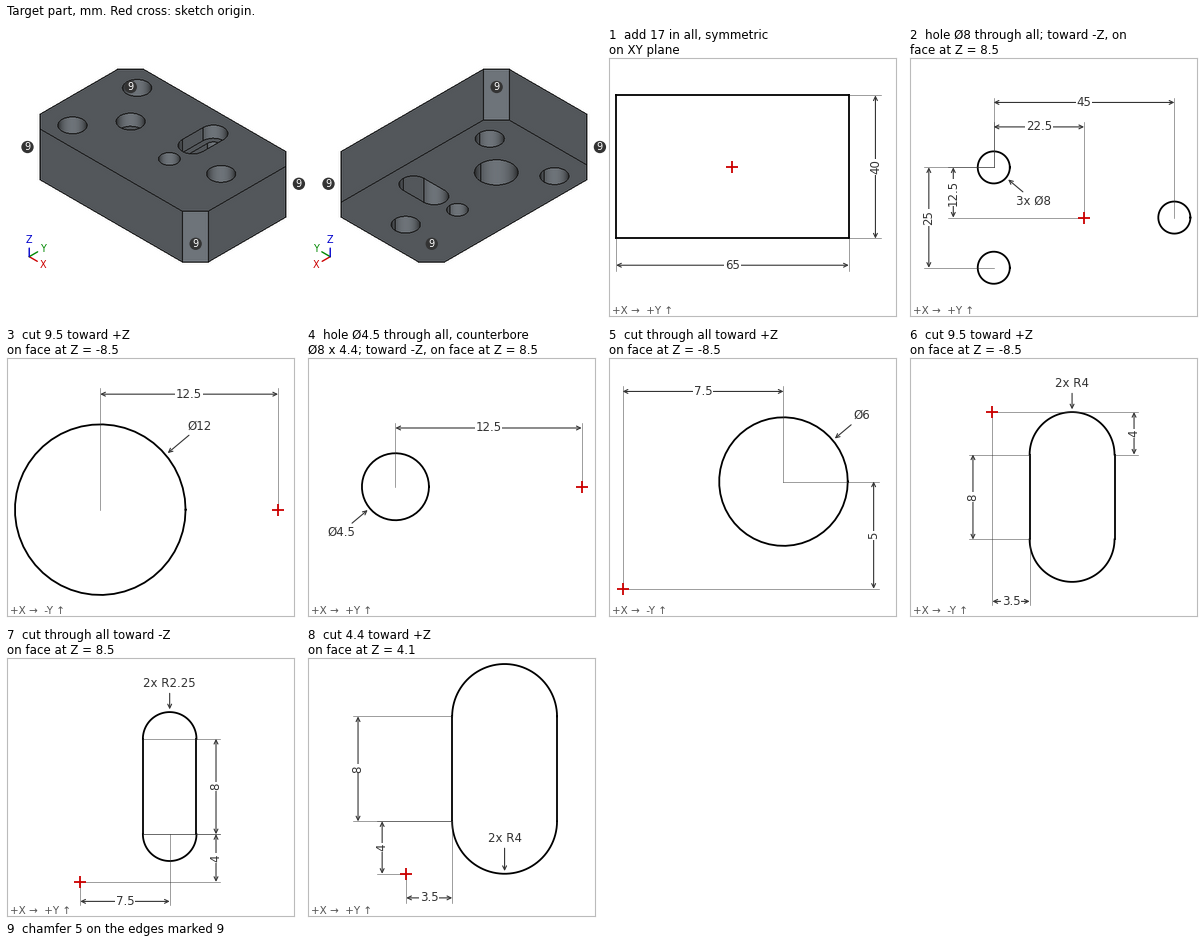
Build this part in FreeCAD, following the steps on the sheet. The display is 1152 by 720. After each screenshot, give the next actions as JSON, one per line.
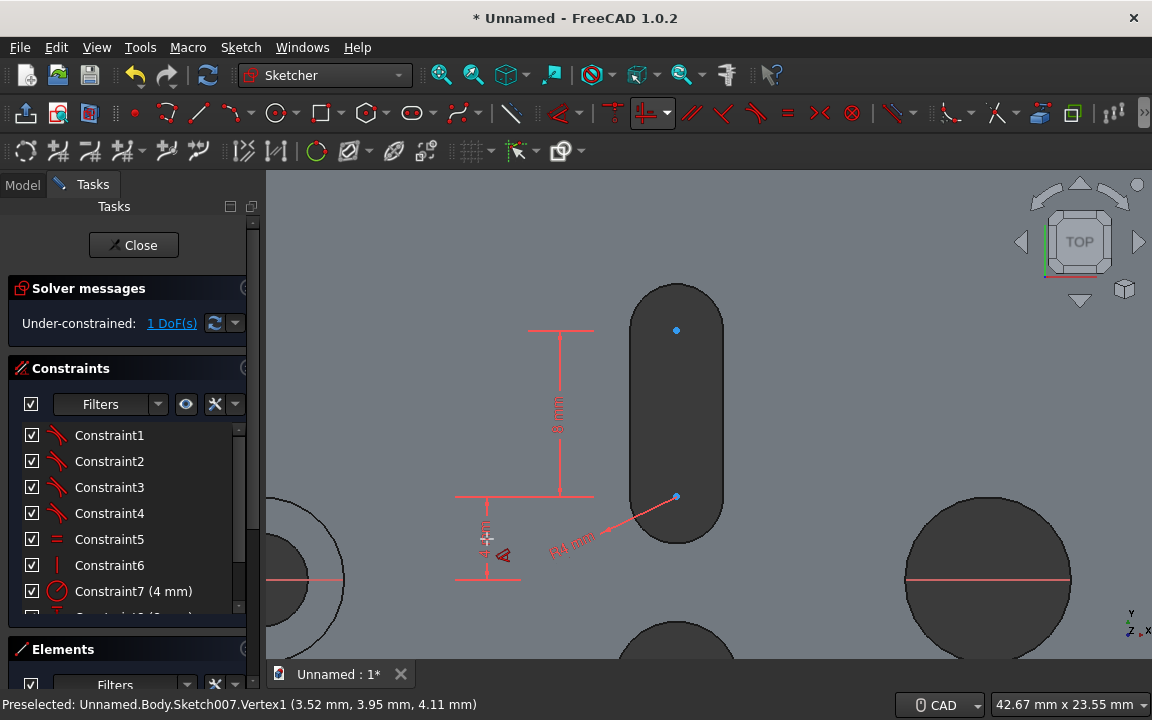
{"action": "left_click", "coordinate": [594, 497]}
{"action": "left_click", "coordinate": [557, 614]}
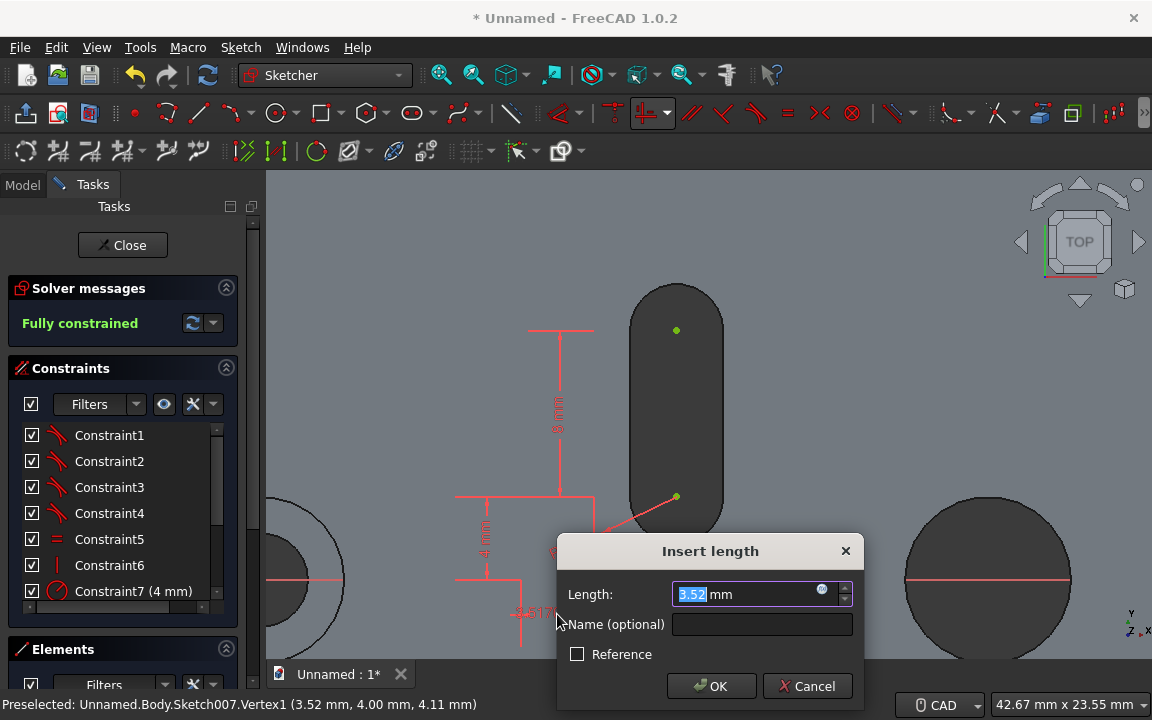
{"action": "type", "text": "3.5"}
{"action": "key", "text": "Return"}
{"action": "key", "text": "Escape"}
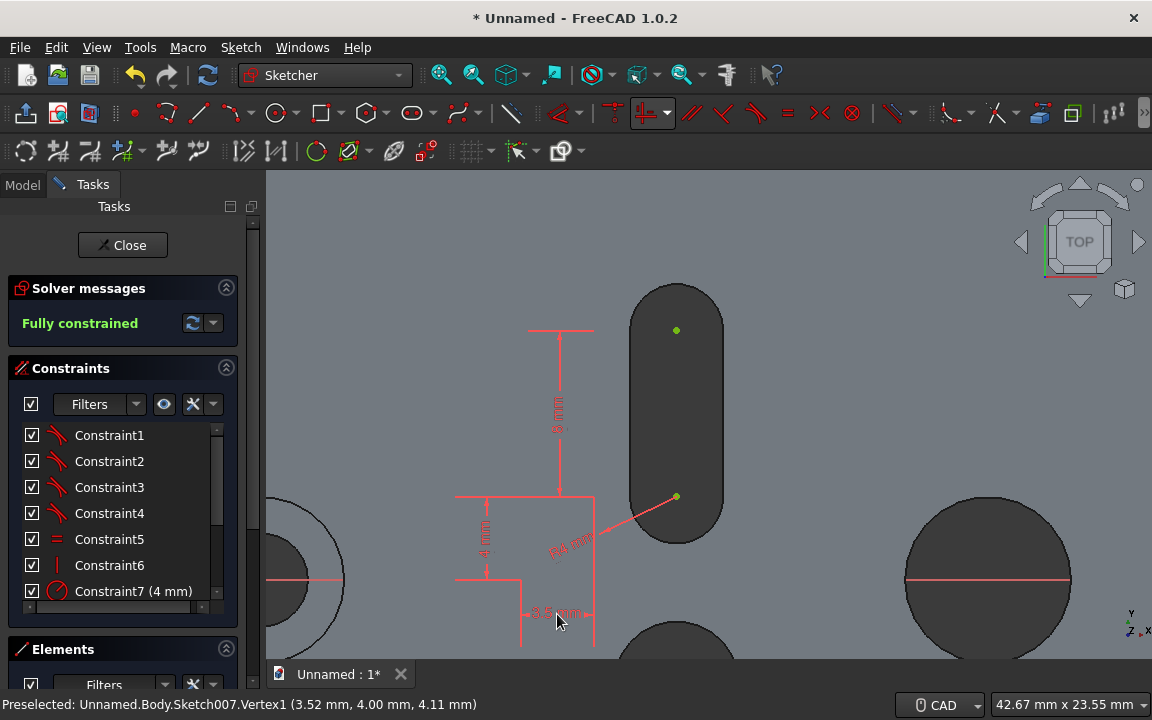
{"action": "left_click", "coordinate": [123, 245]}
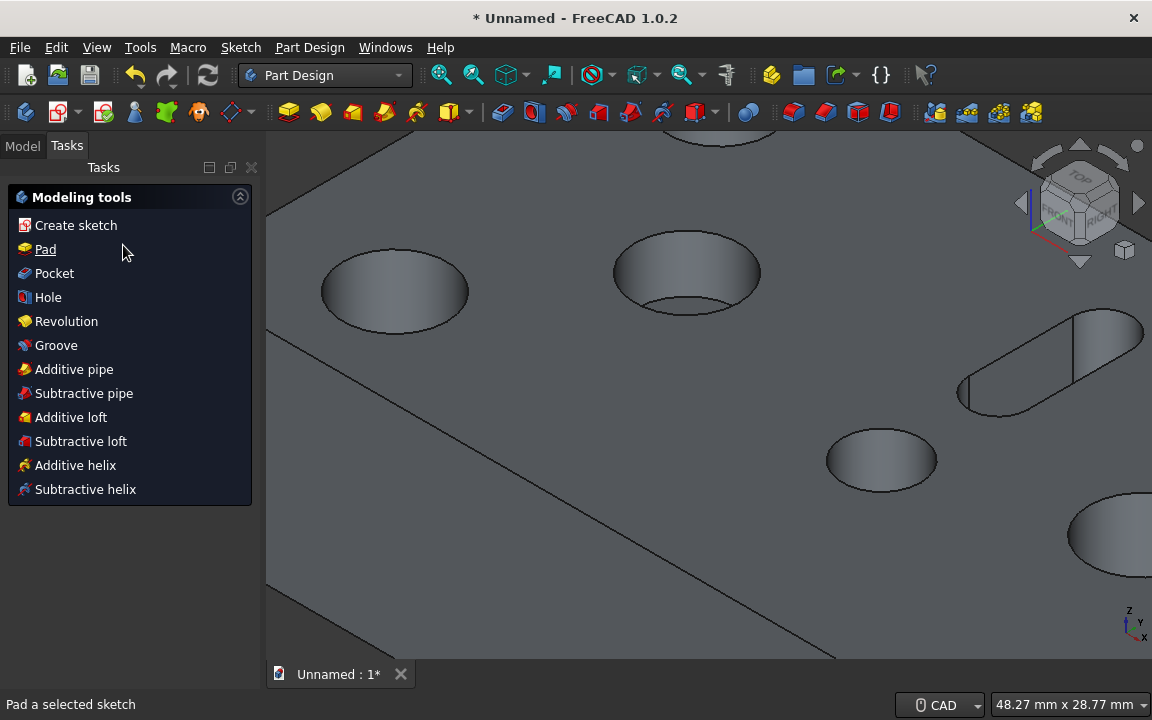
{"action": "left_click", "coordinate": [504, 112]}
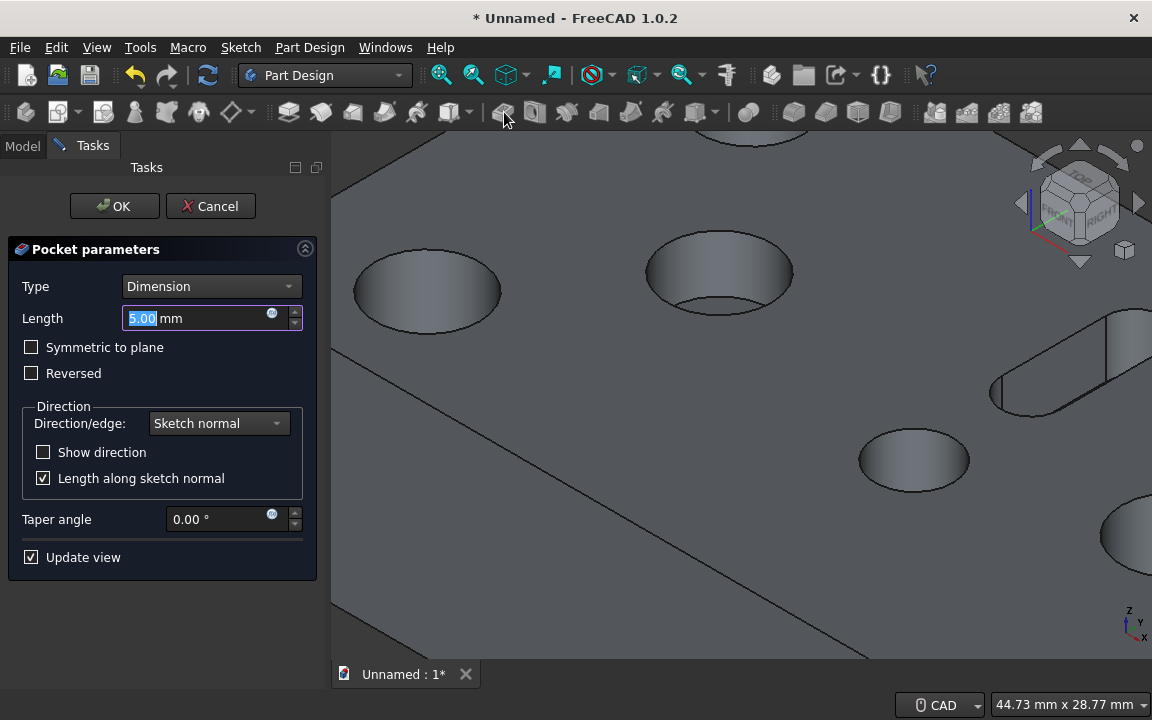
{"action": "type", "text": "4.4"}
{"action": "key", "text": "Tab"}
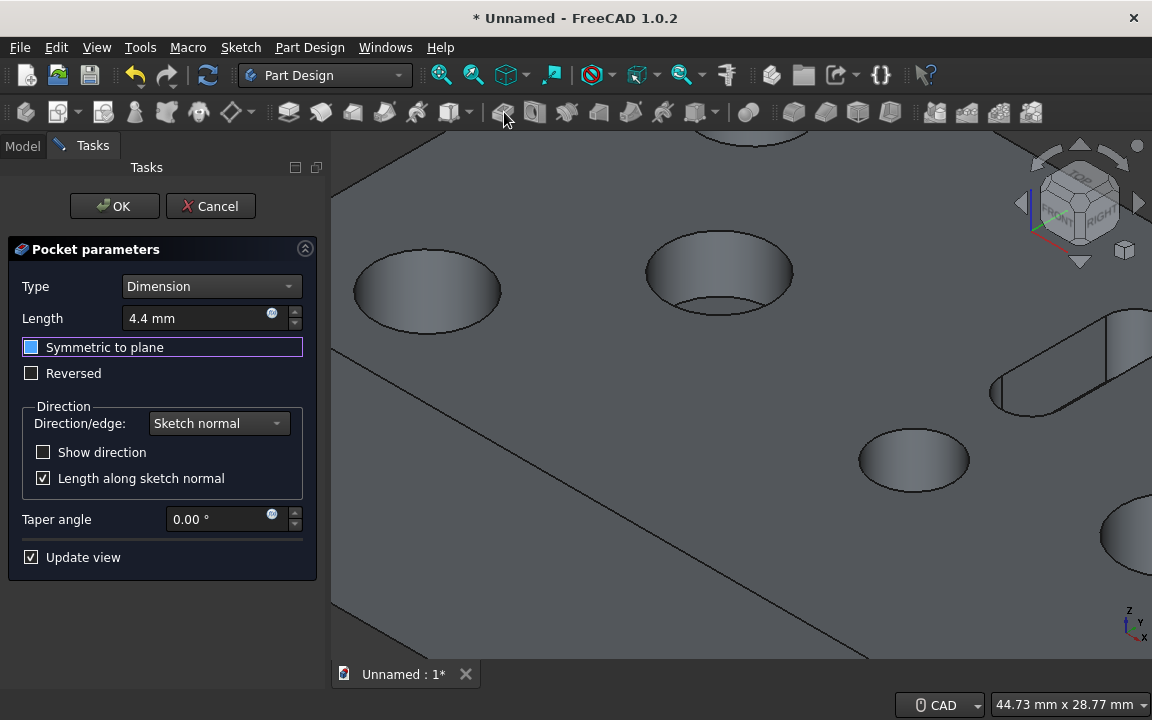
{"action": "left_click", "coordinate": [30, 373]}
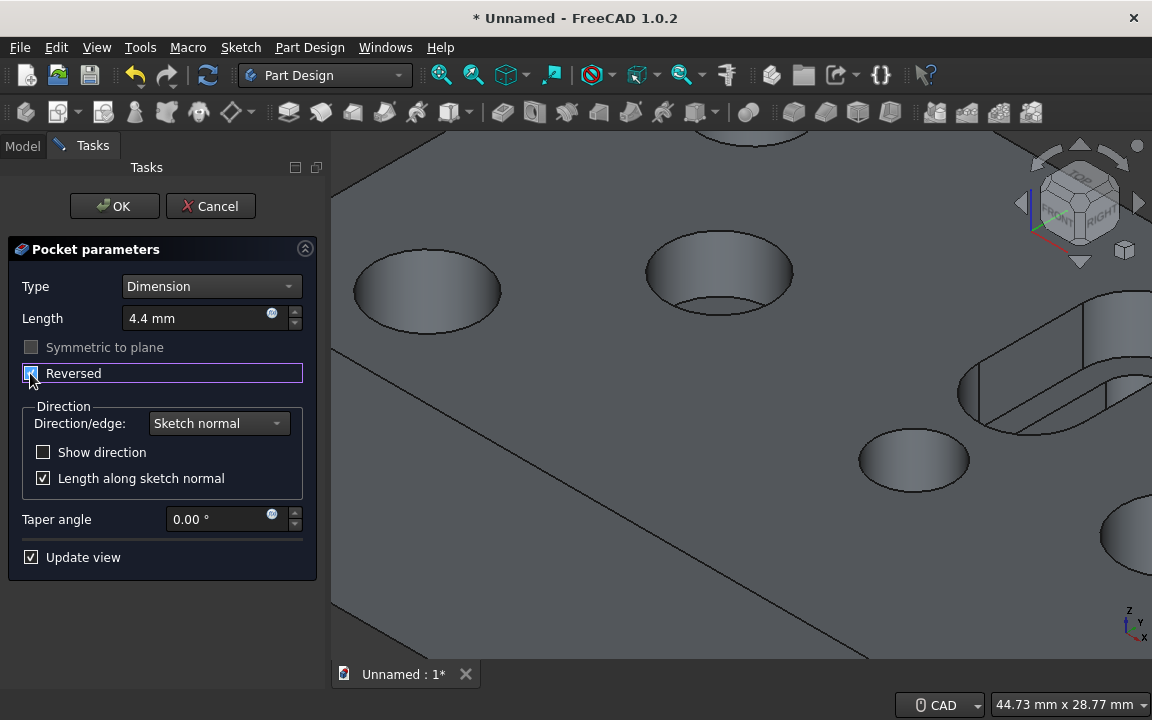
{"action": "left_click", "coordinate": [115, 206]}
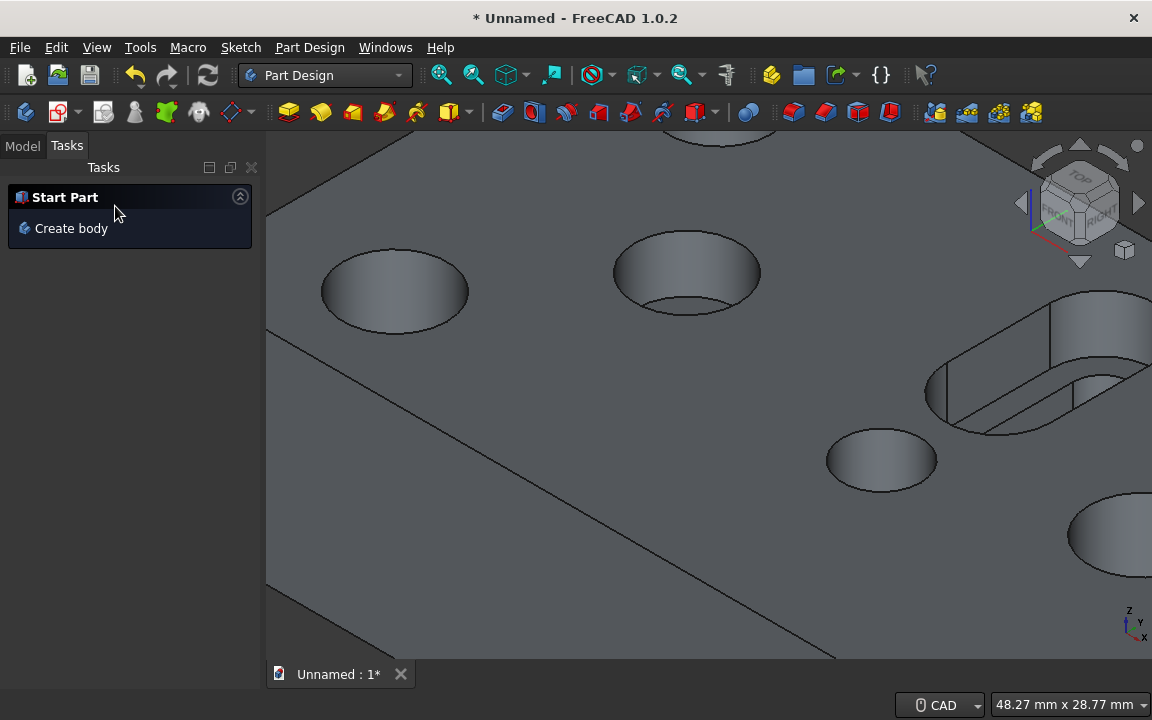
{"action": "left_click", "coordinate": [442, 76]}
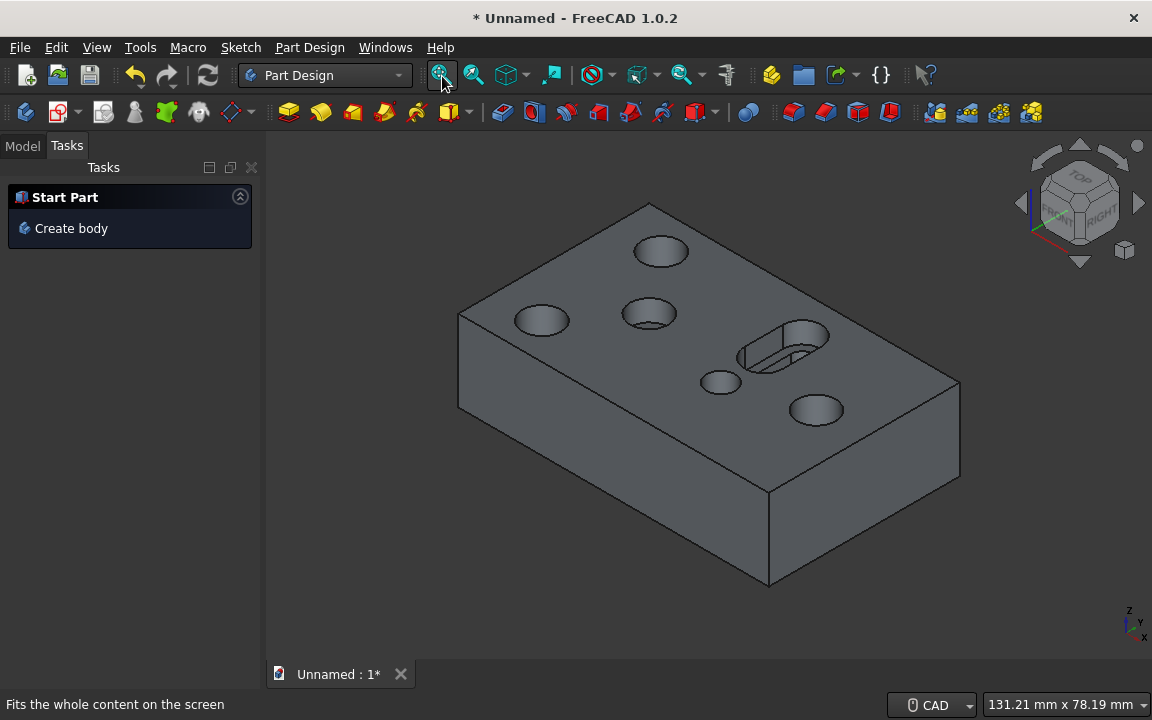
{"action": "left_click", "coordinate": [769, 539]}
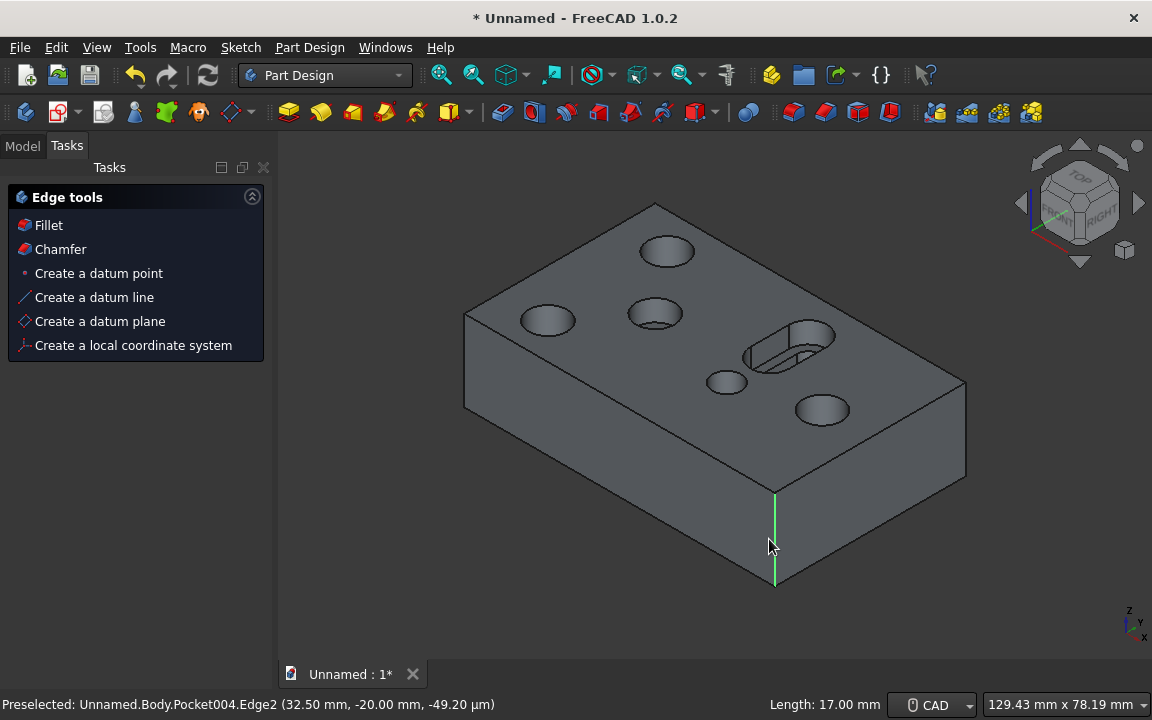
{"action": "key", "text": "2"}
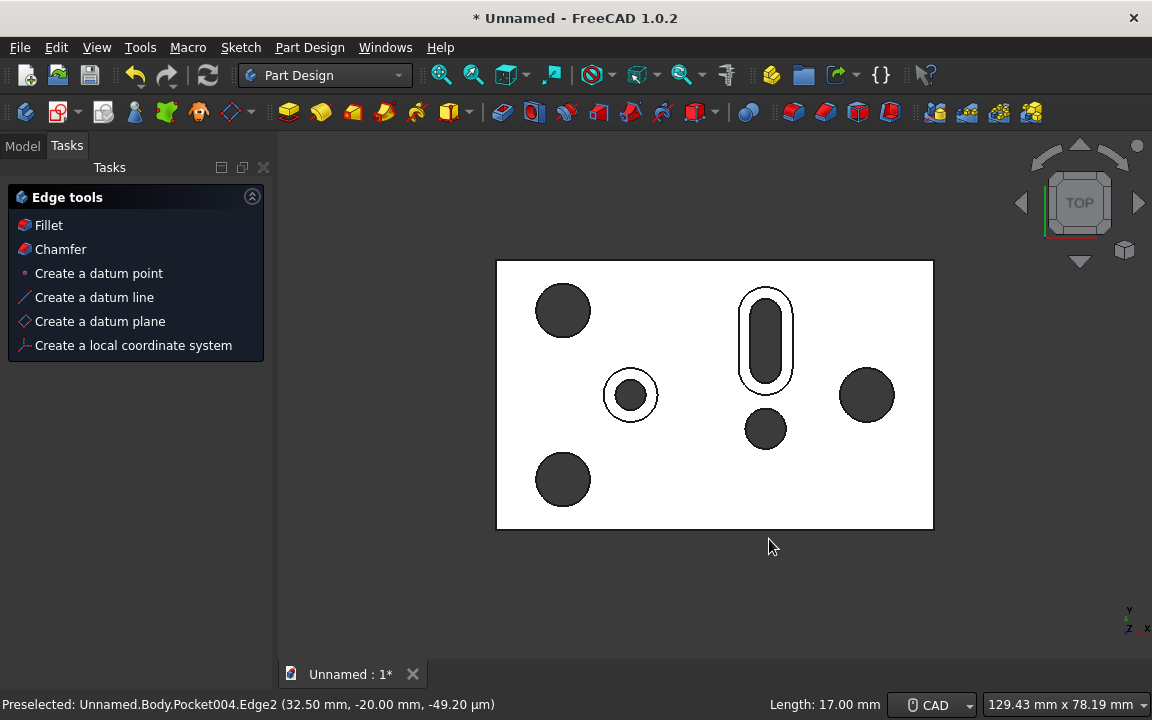
{"action": "key", "text": "0"}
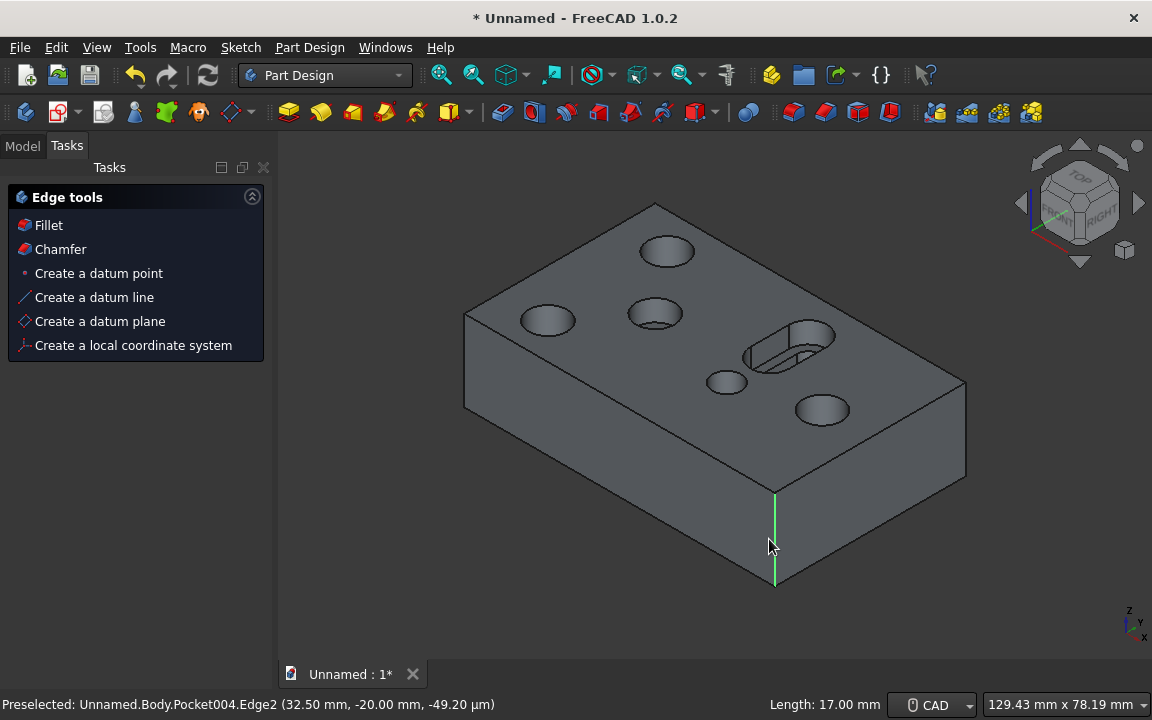
{"action": "key", "text": "1"}